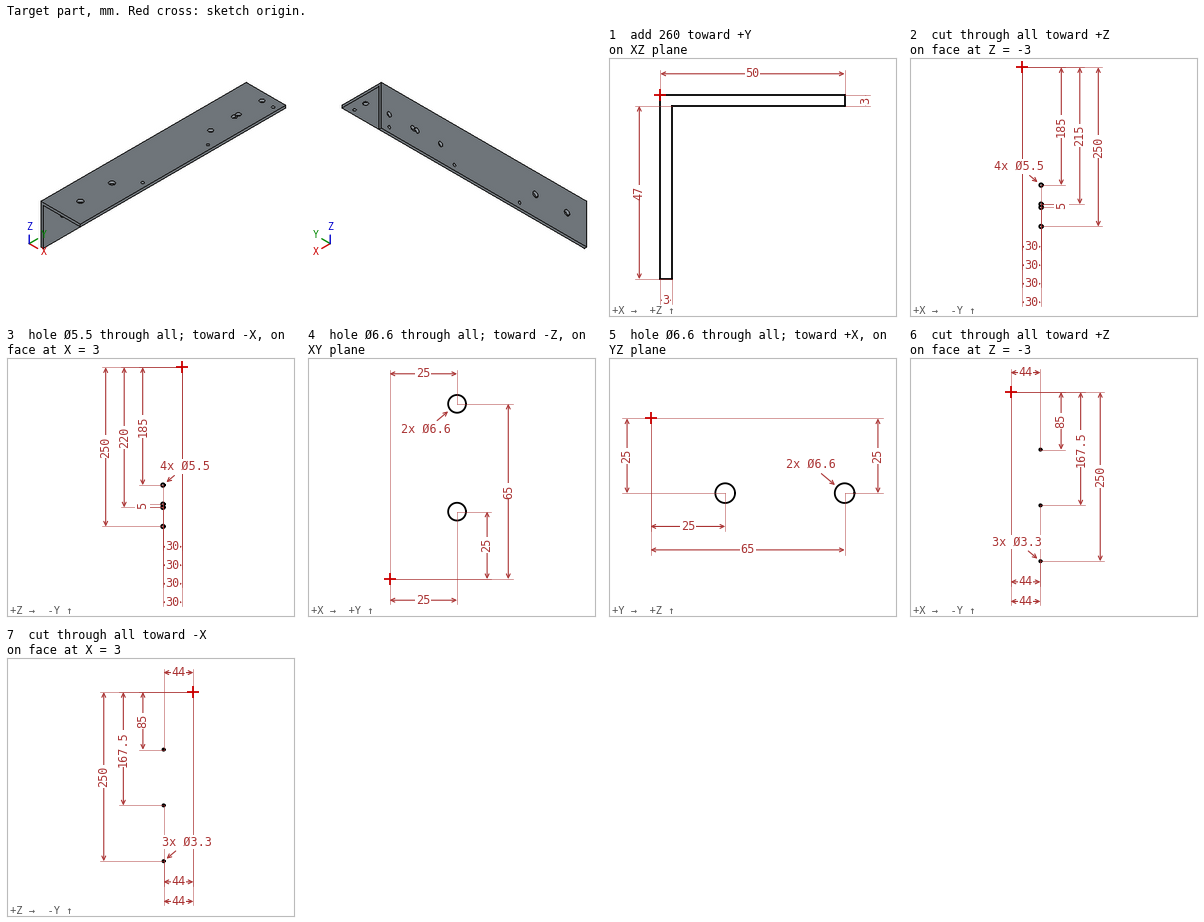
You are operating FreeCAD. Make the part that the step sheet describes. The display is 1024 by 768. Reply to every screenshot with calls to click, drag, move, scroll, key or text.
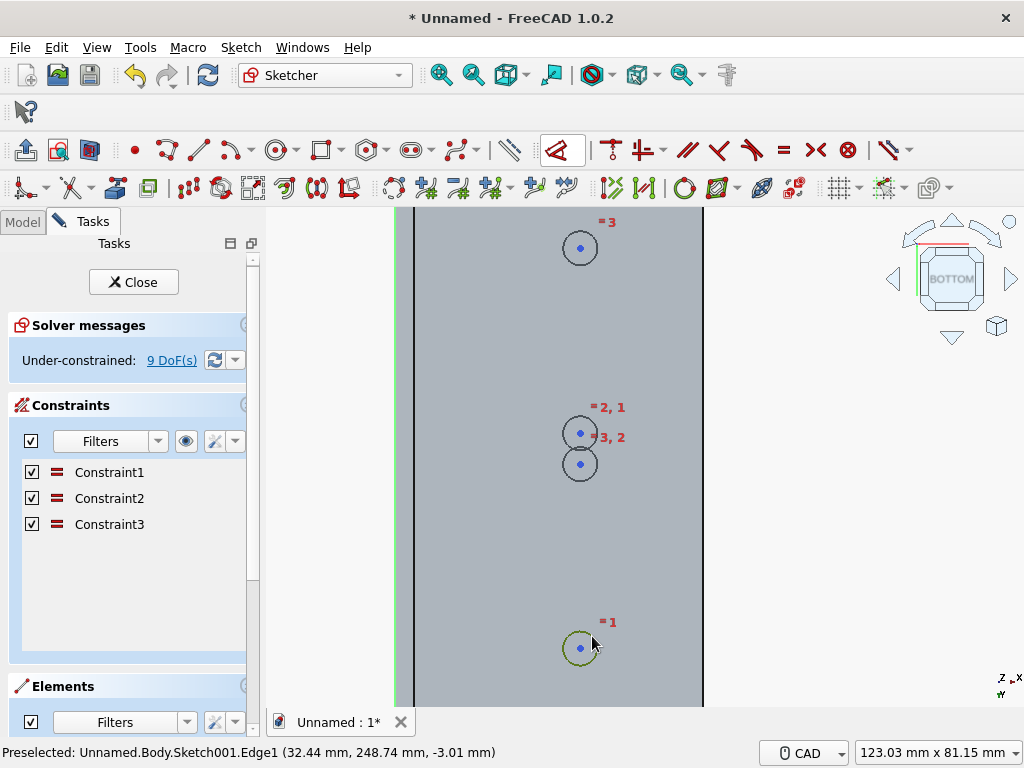
key(k)
key(o)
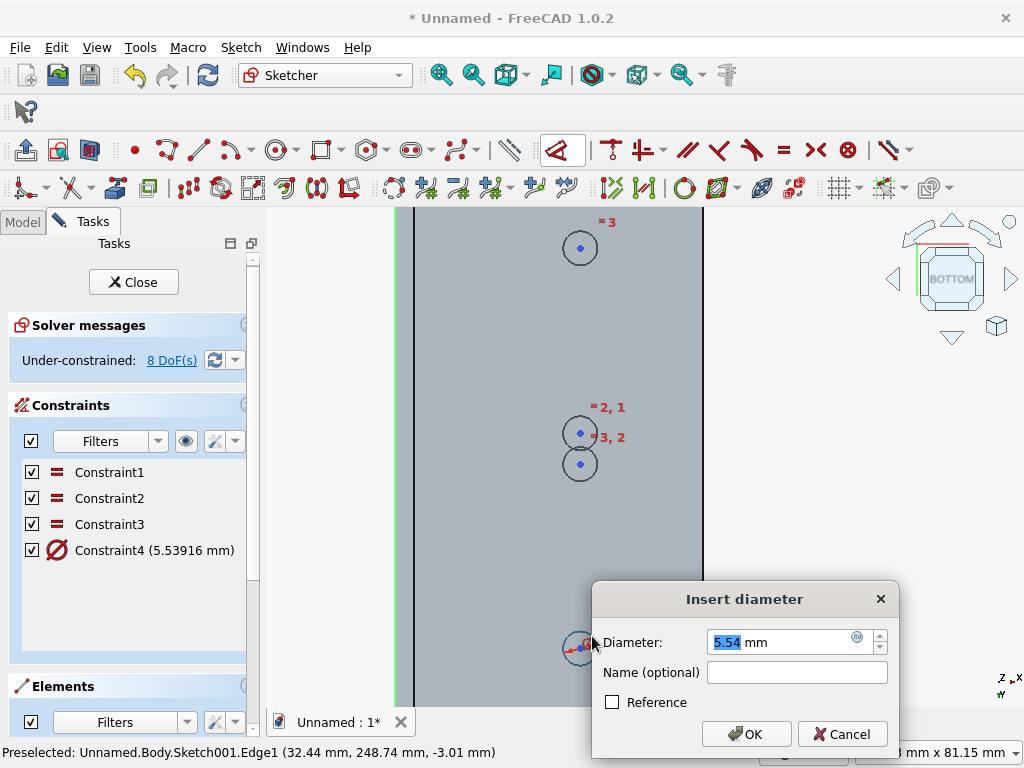
text(5.5)
key(Return)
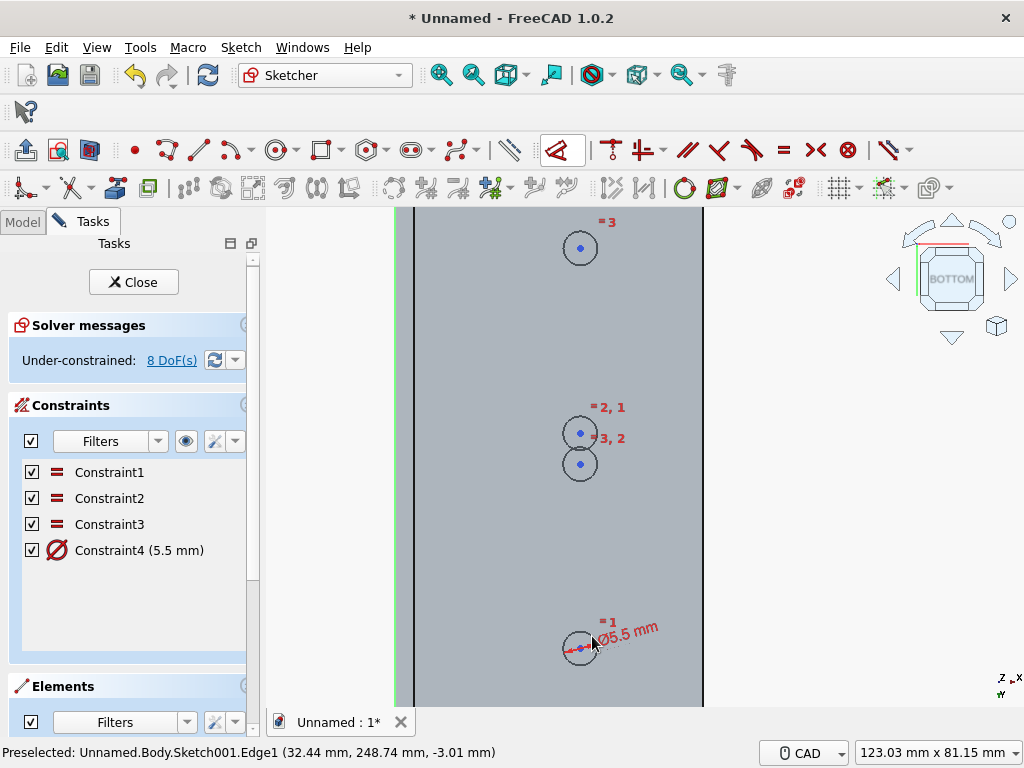
click(580, 649)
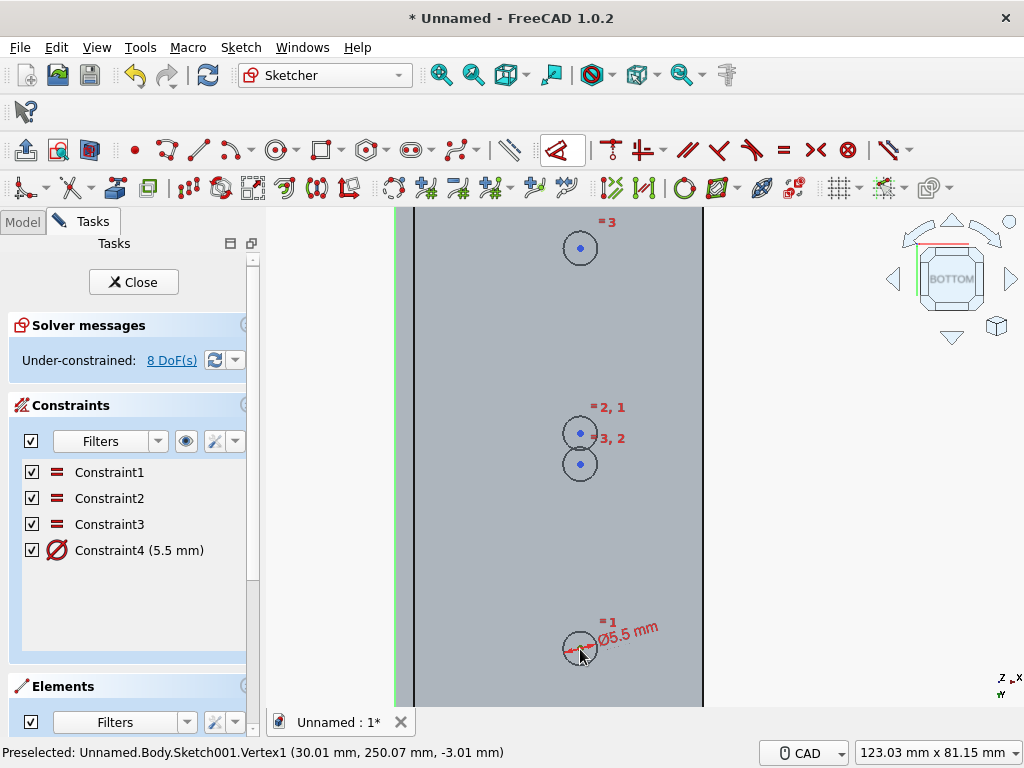
key(l)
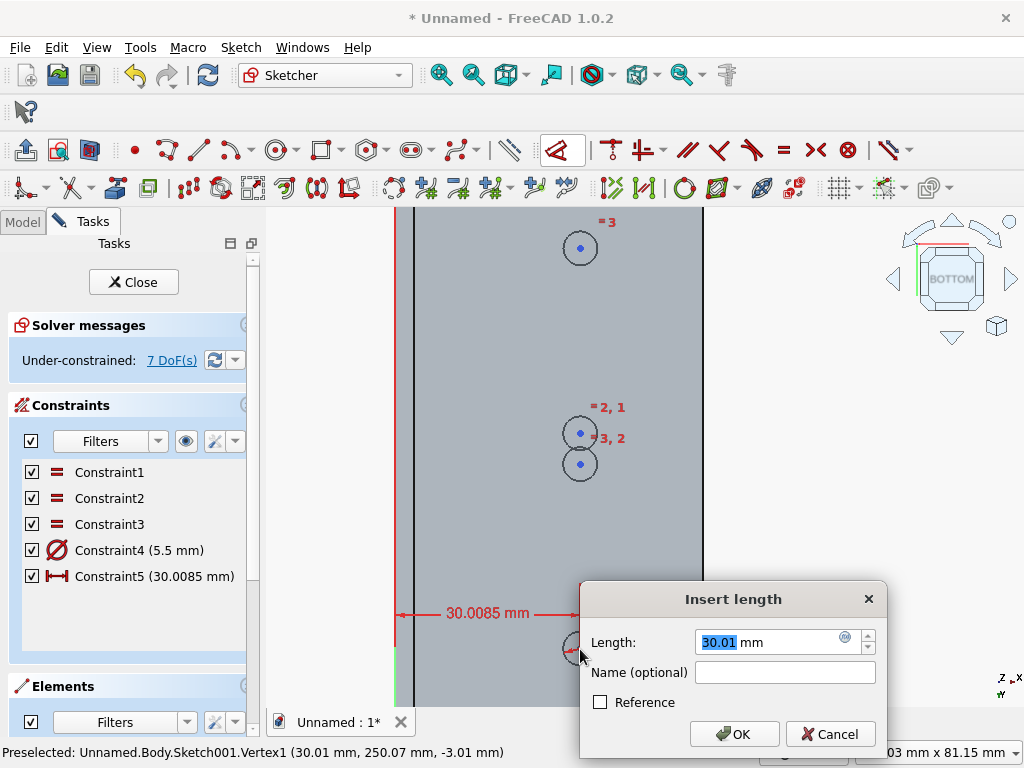
text(30)
key(Return)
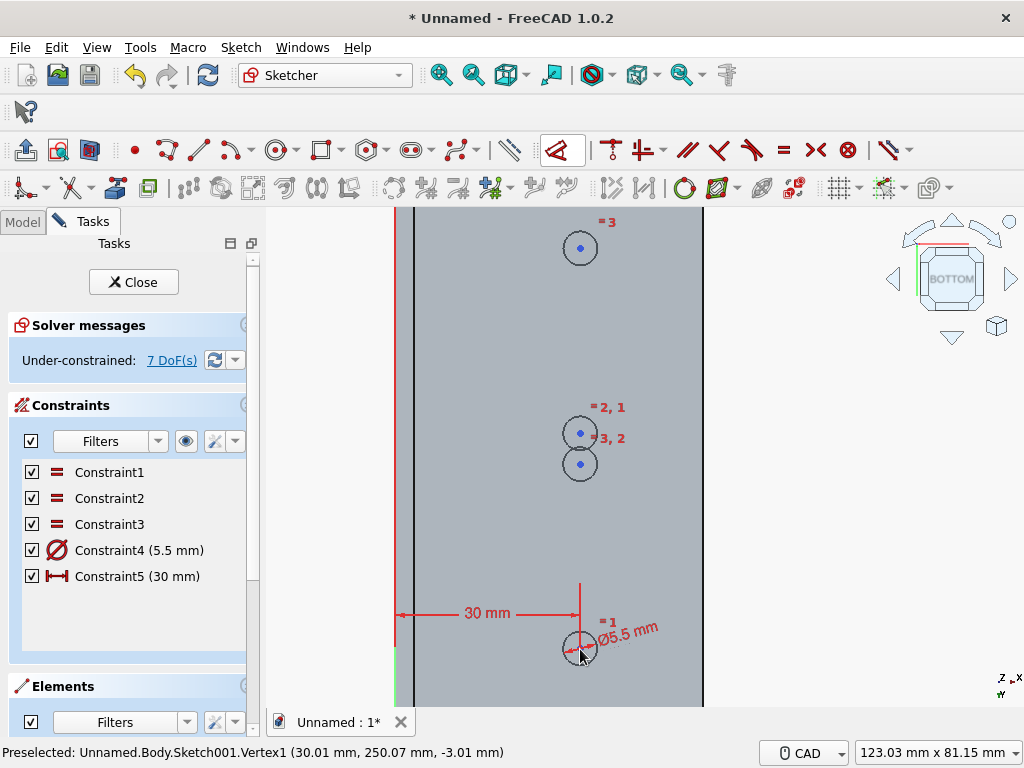
click(580, 433)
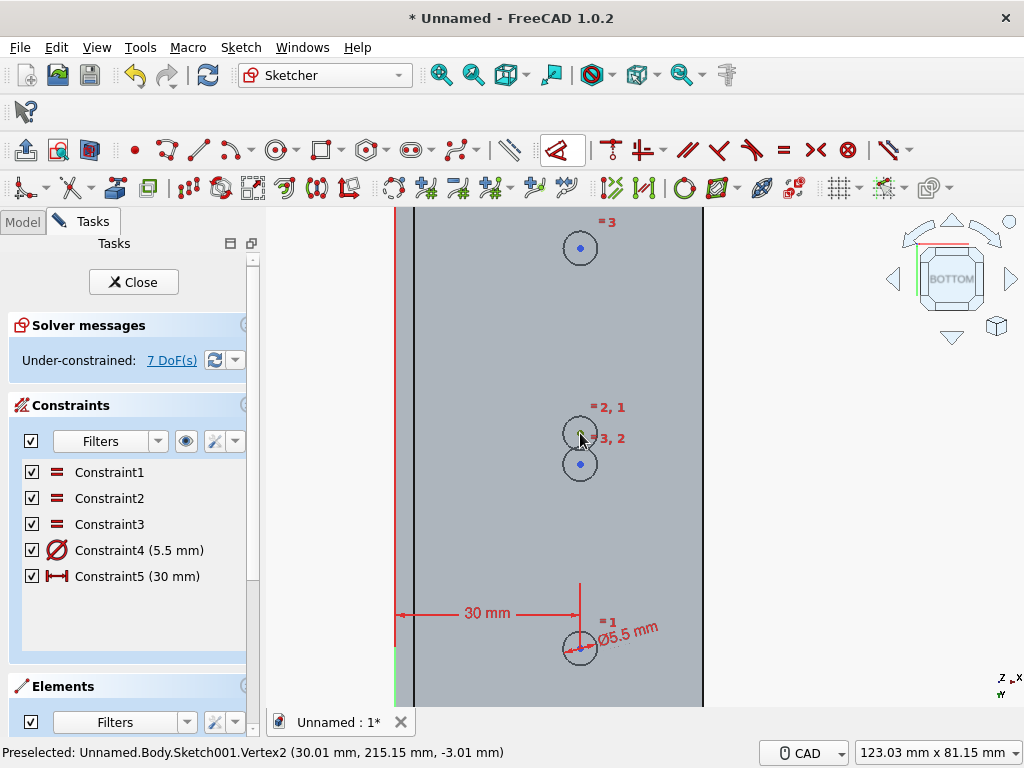
key(l)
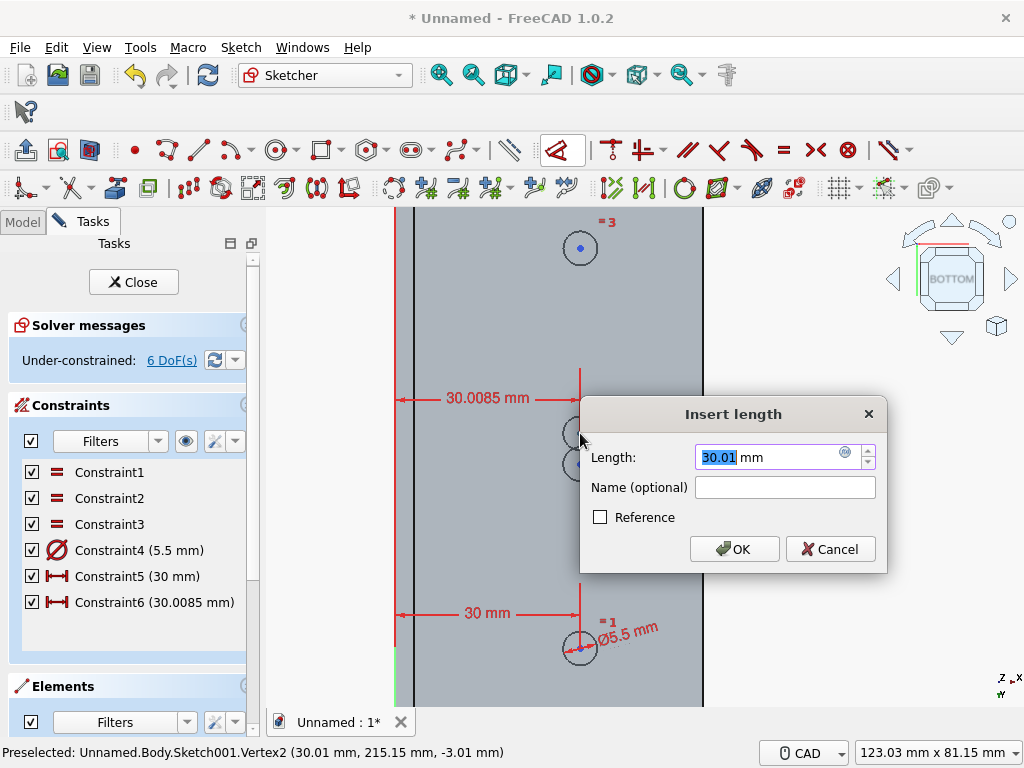
text(30)
key(Return)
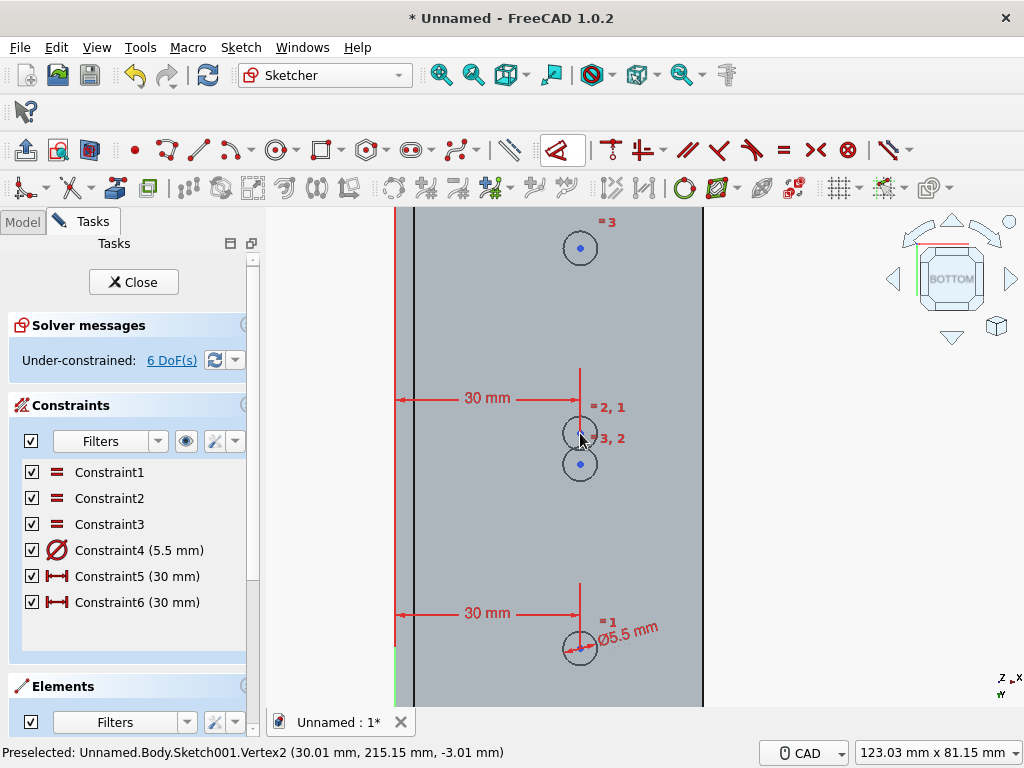
click(580, 464)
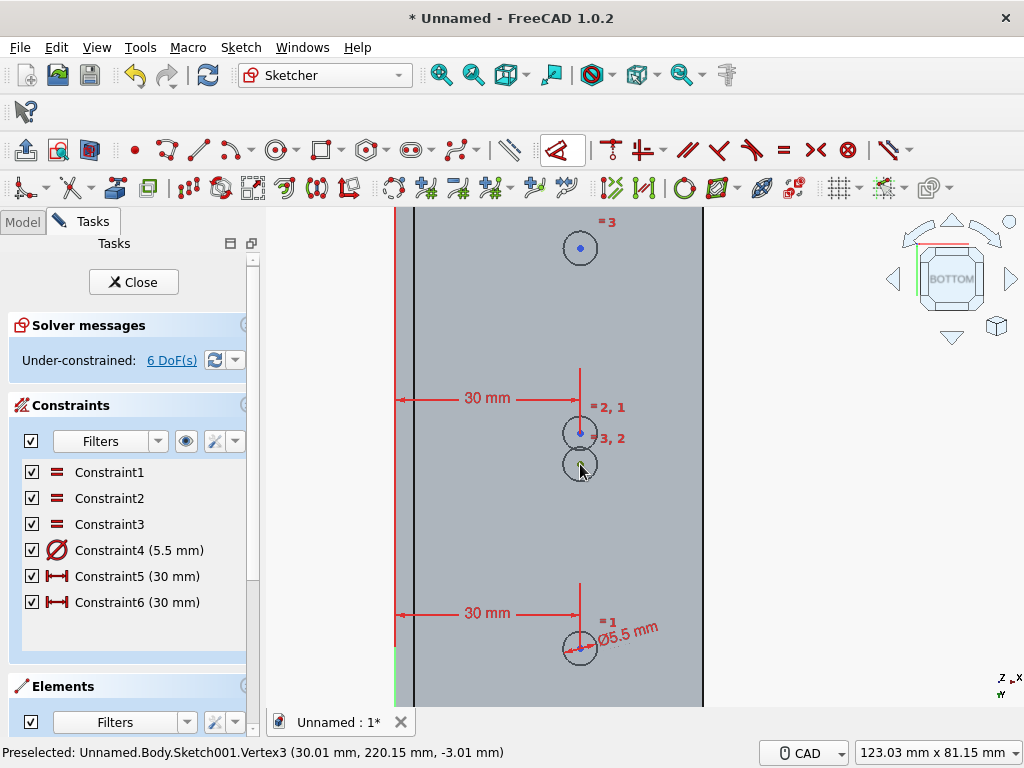
key(l)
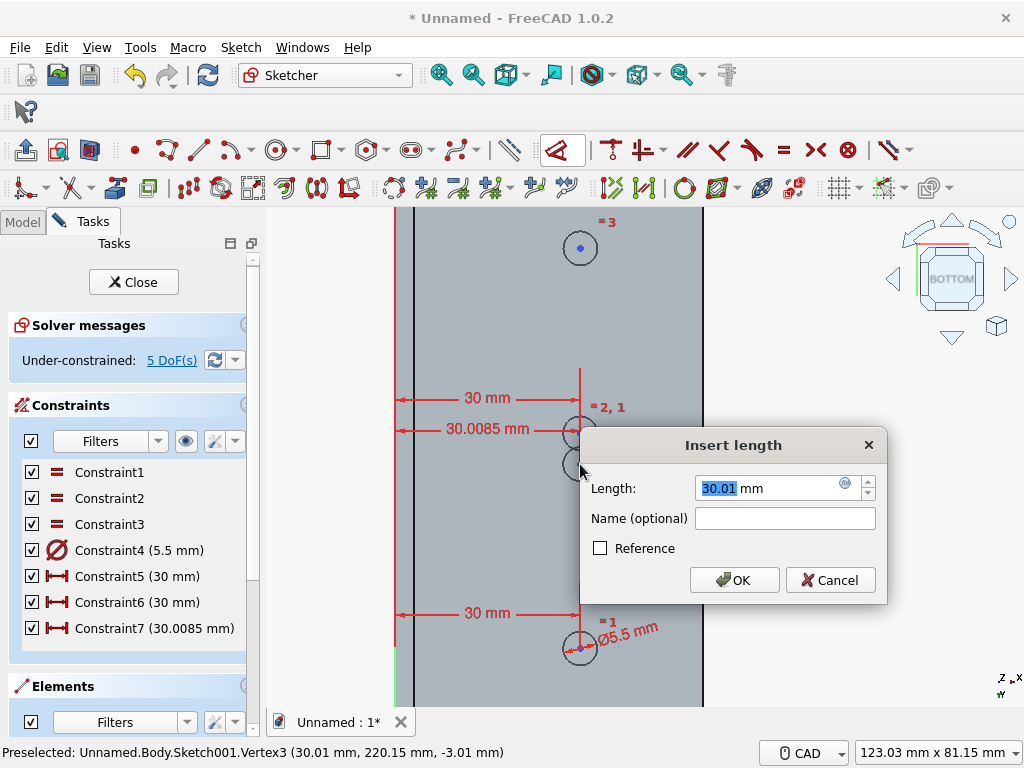
text(30)
key(Return)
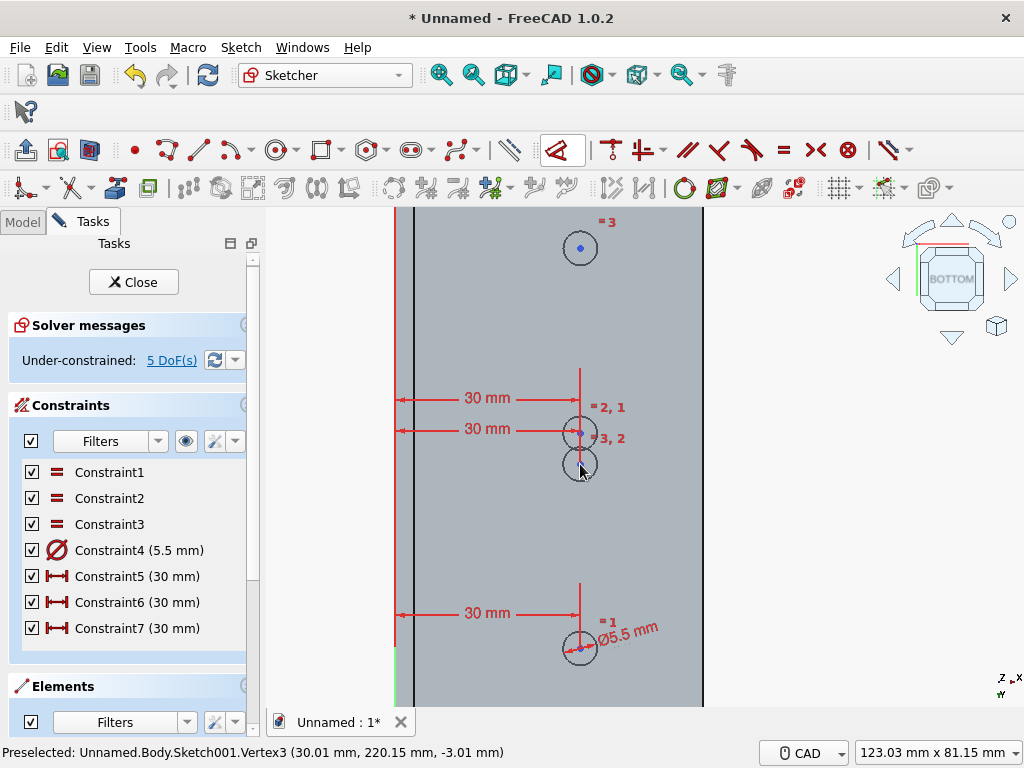
click(580, 248)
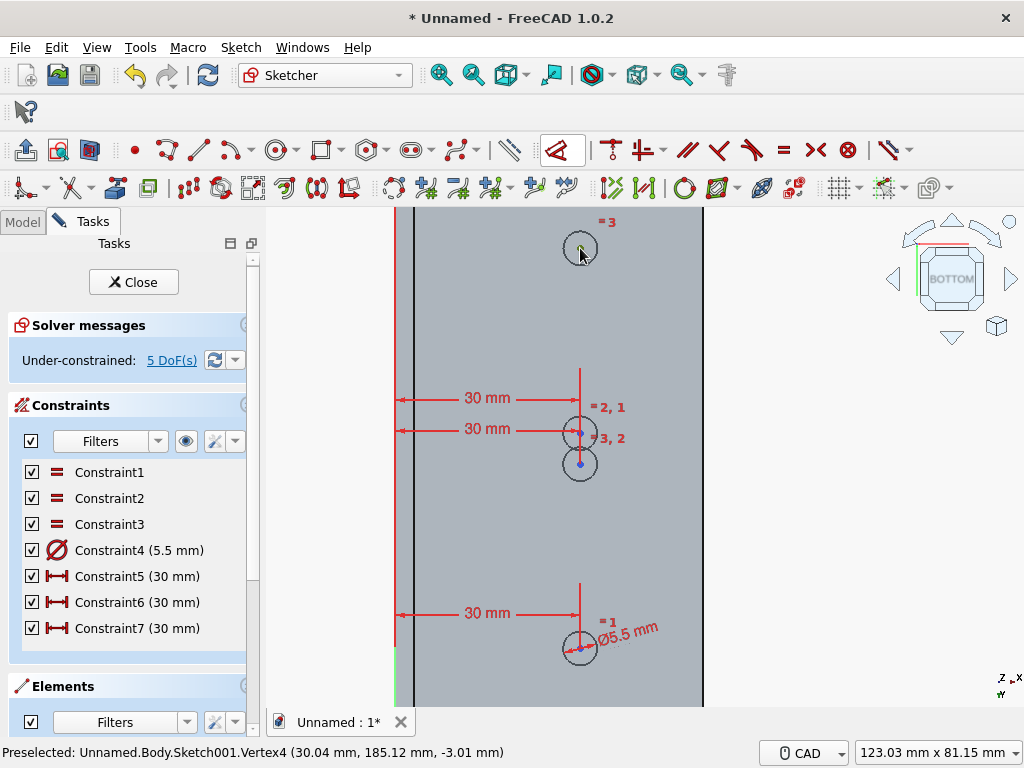
key(l)